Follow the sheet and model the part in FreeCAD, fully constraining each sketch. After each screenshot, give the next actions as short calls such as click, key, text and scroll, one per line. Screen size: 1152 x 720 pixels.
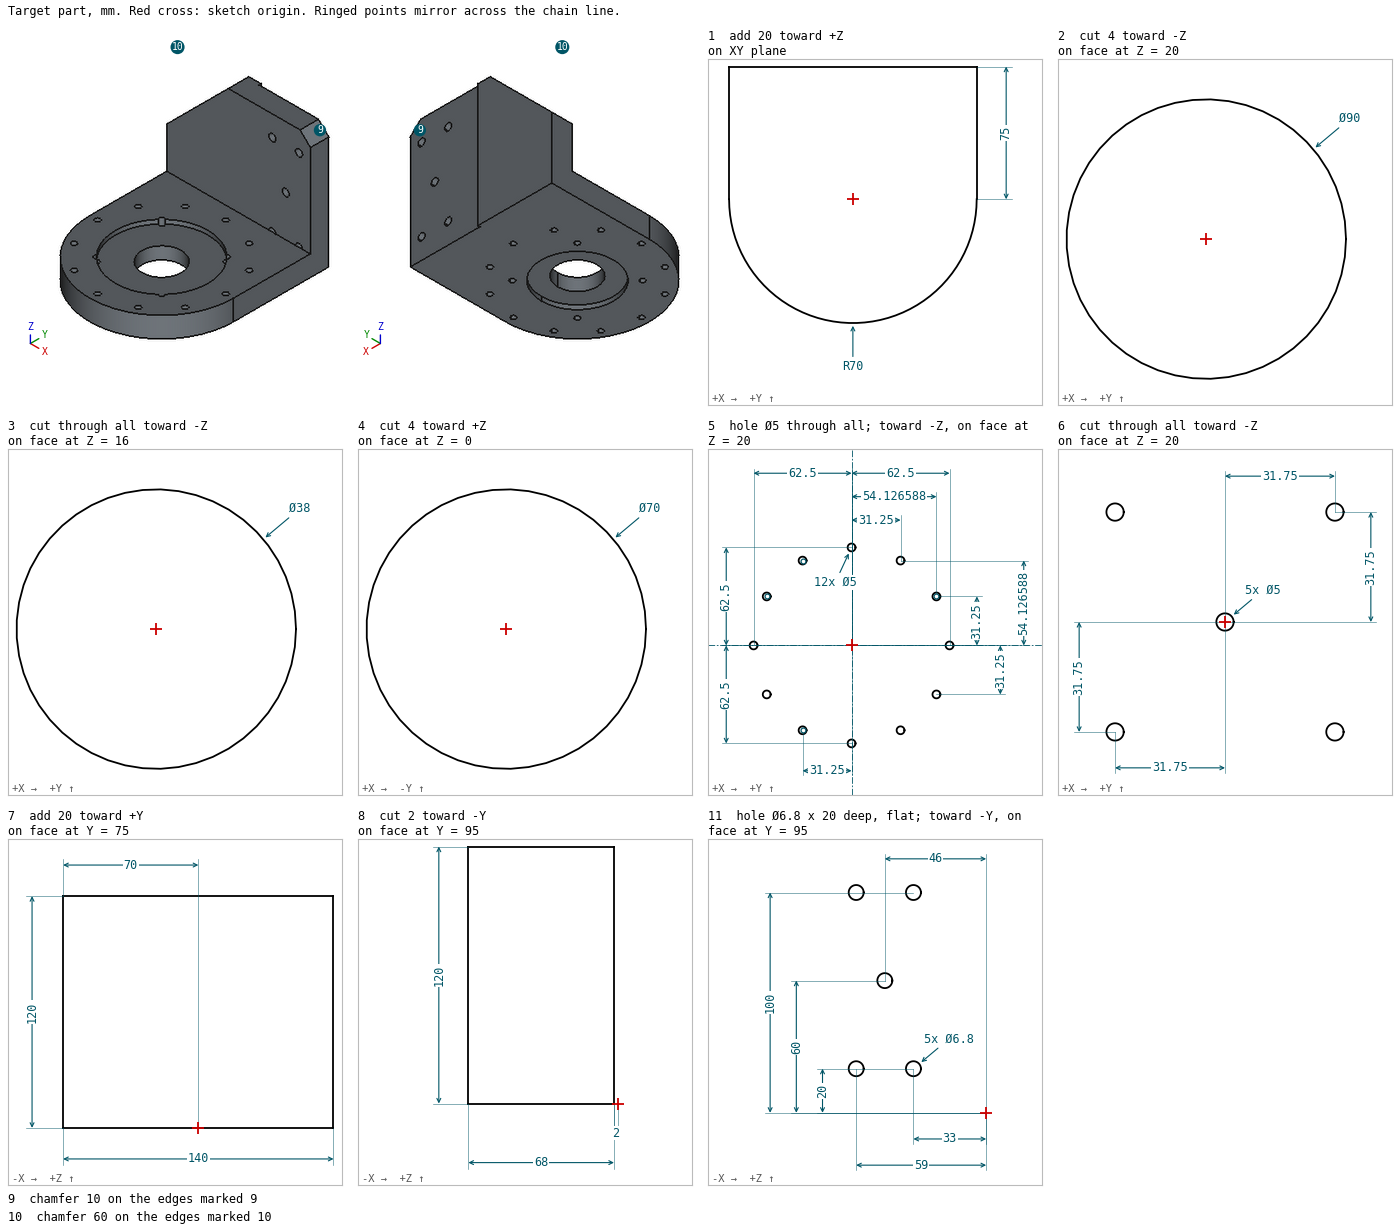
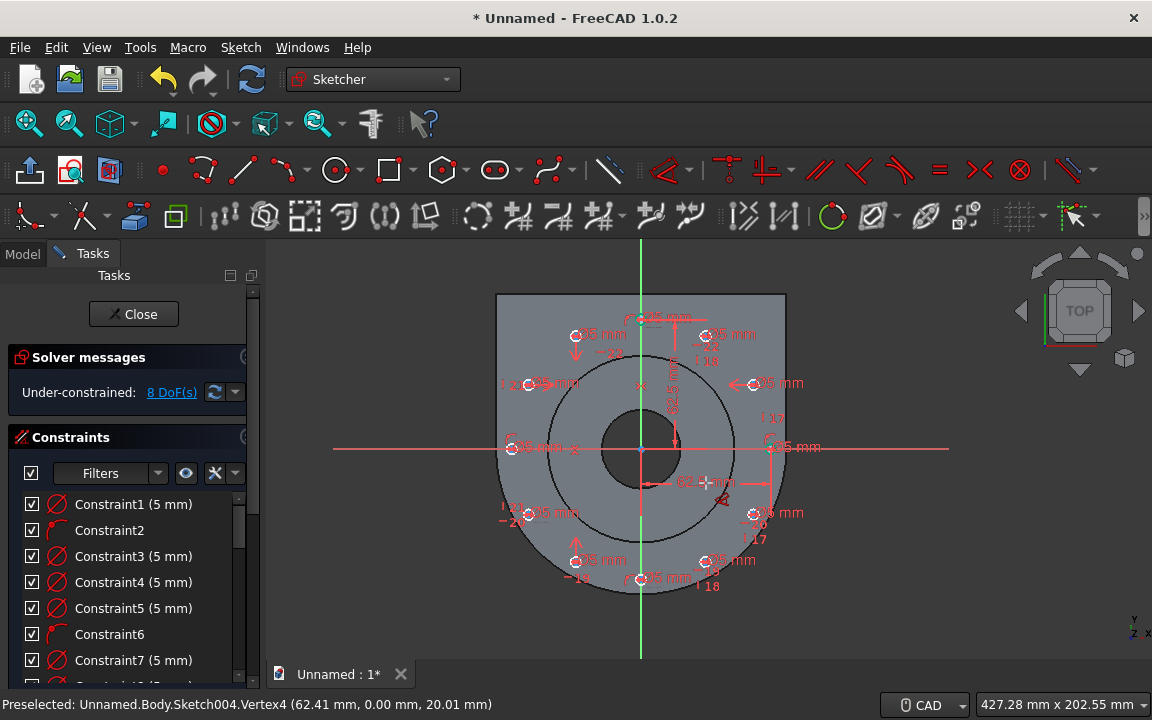
click(641, 580)
click(675, 514)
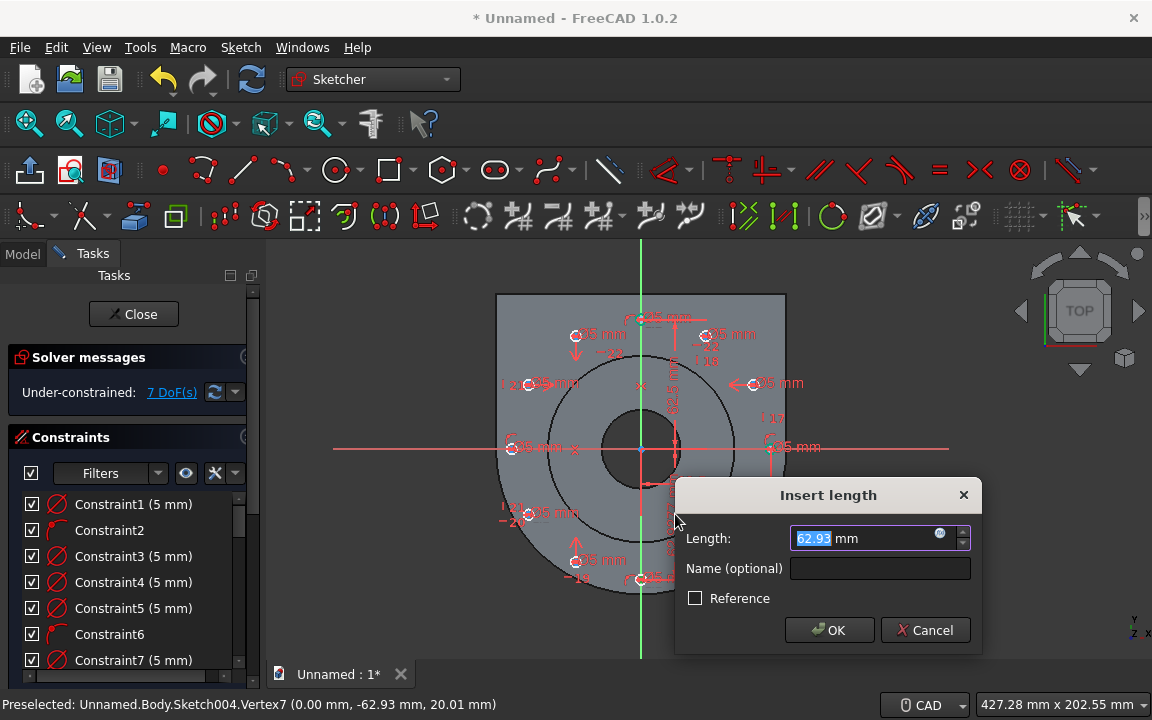
text(62.5)
key(Return)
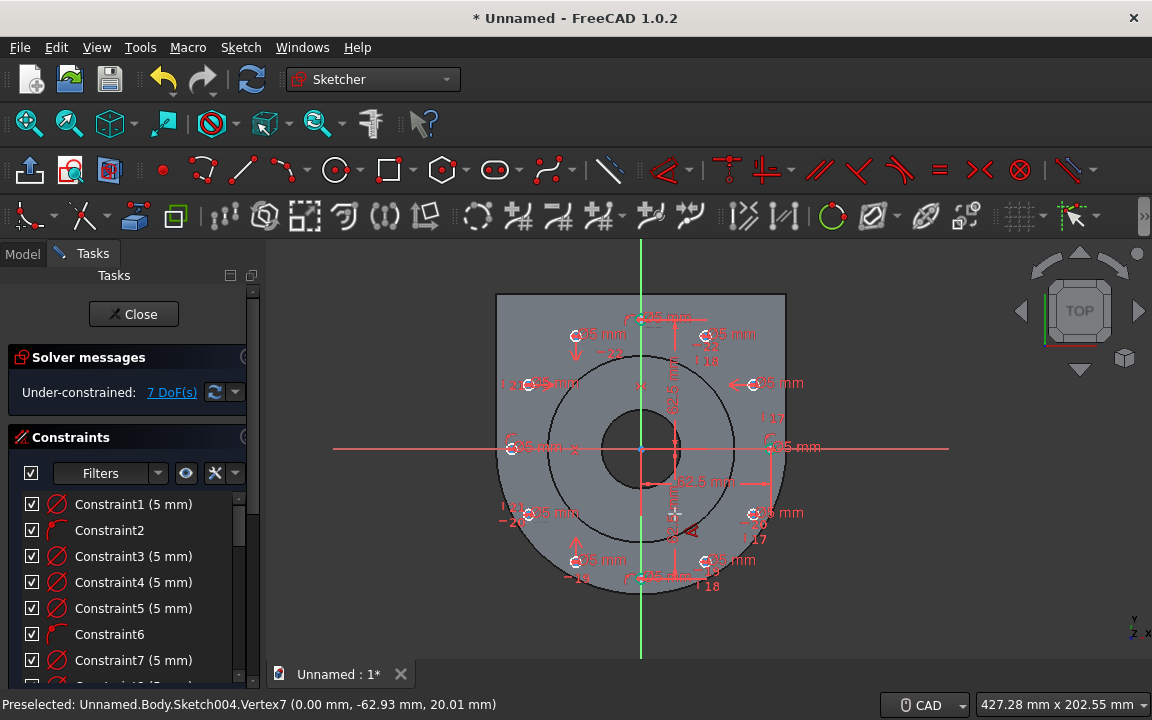
click(512, 449)
click(576, 483)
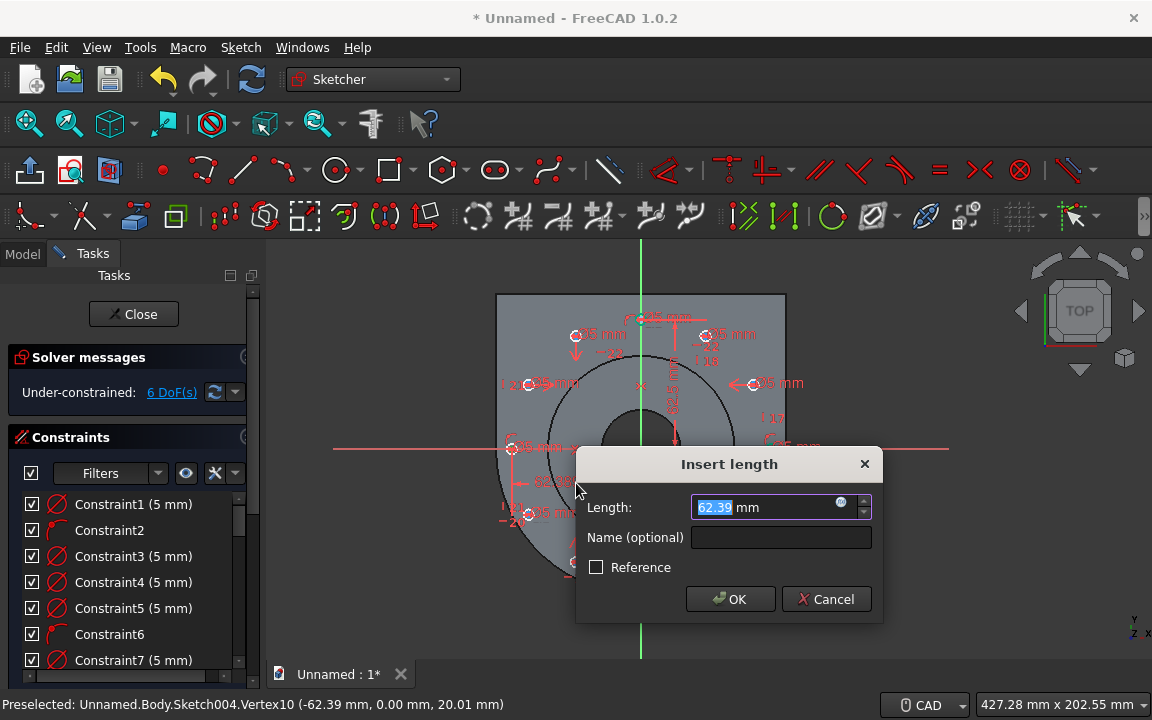
text(62.5)
key(Return)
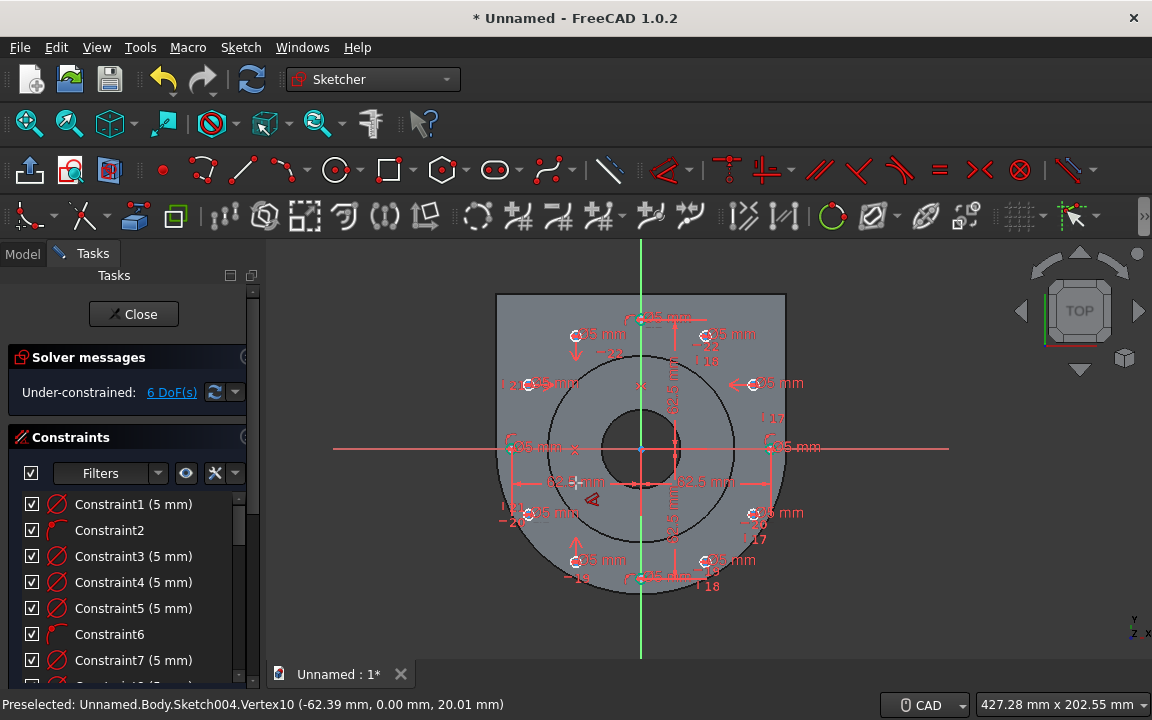
click(706, 336)
click(673, 302)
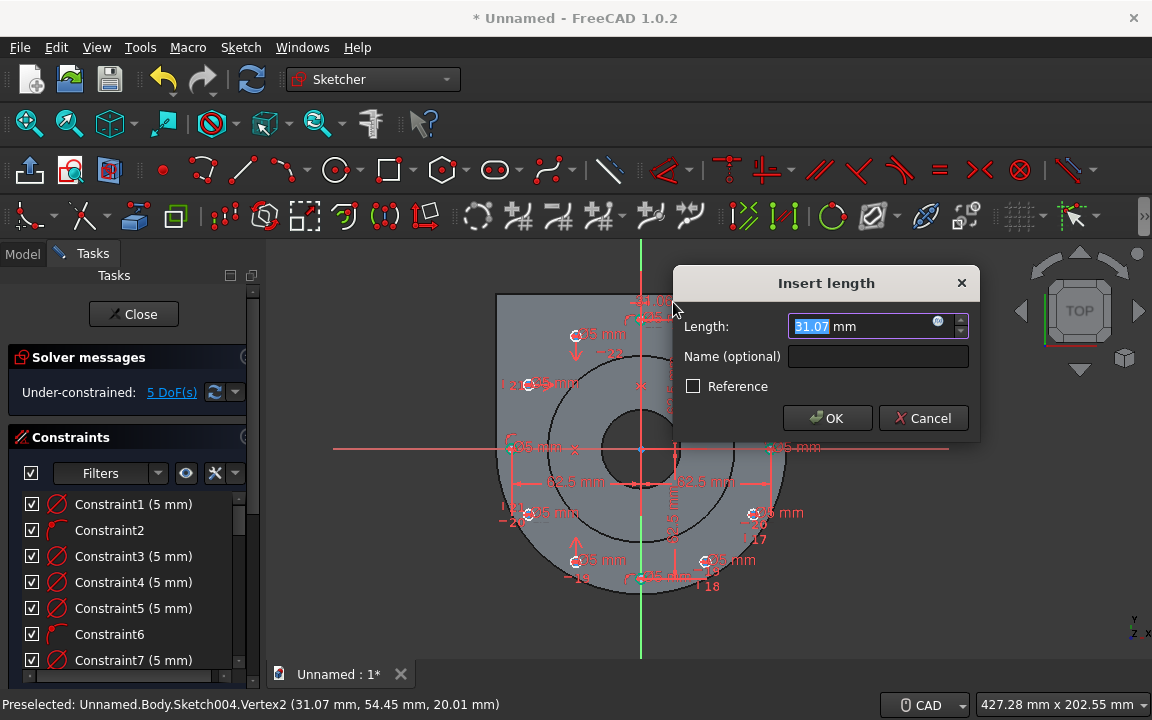
text(31.25)
key(Return)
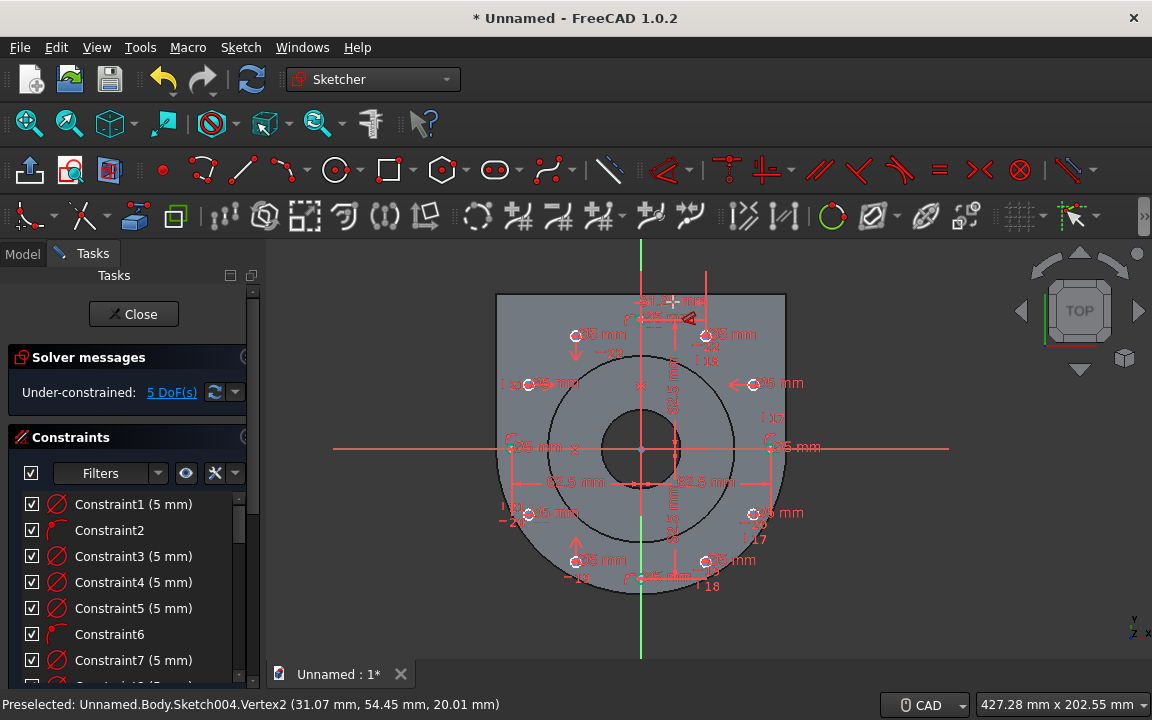
click(754, 385)
click(788, 417)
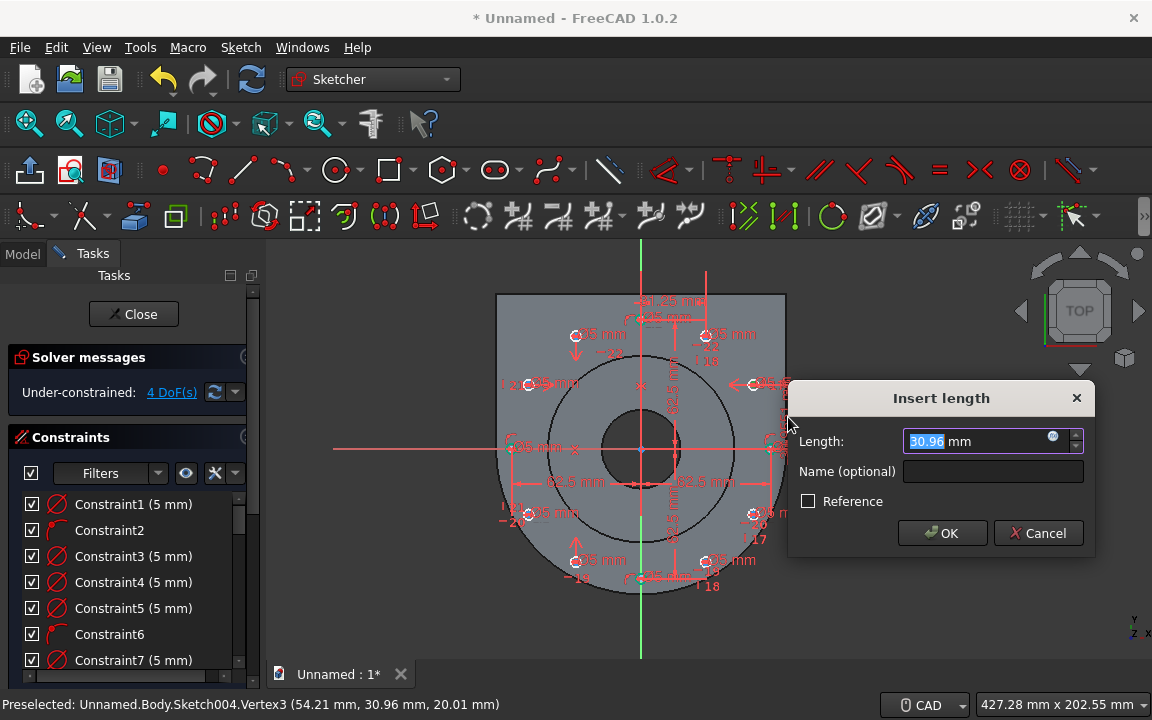
text(31.25)
key(Return)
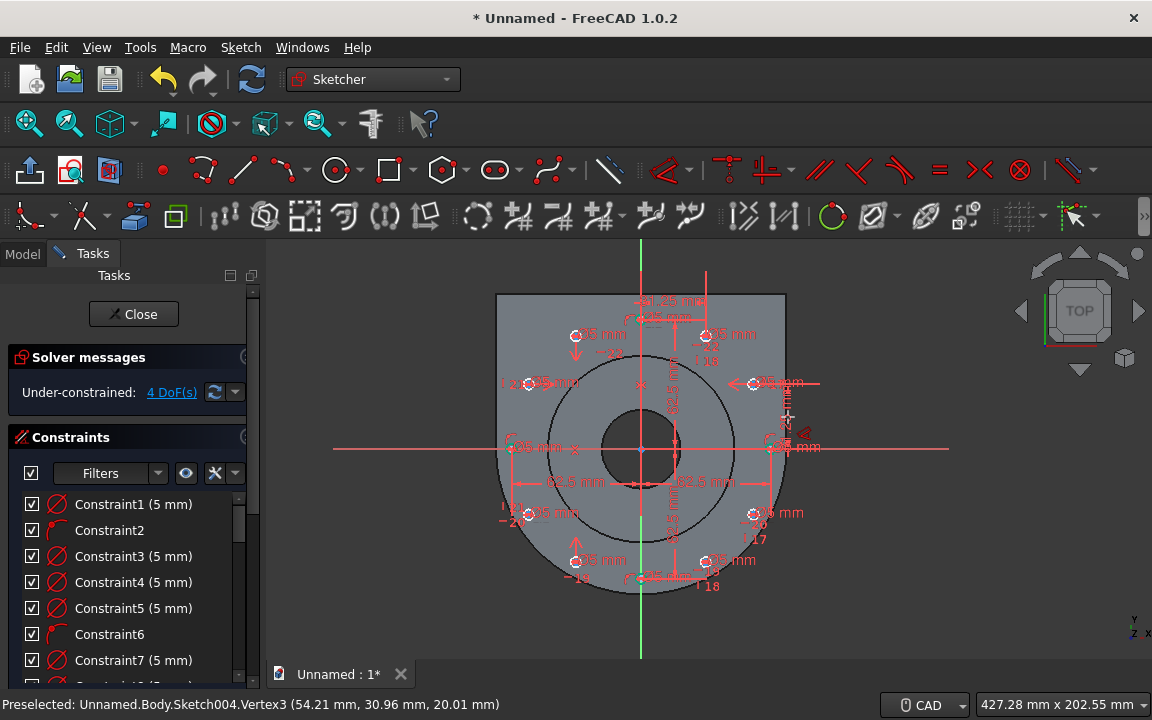
click(754, 515)
click(788, 482)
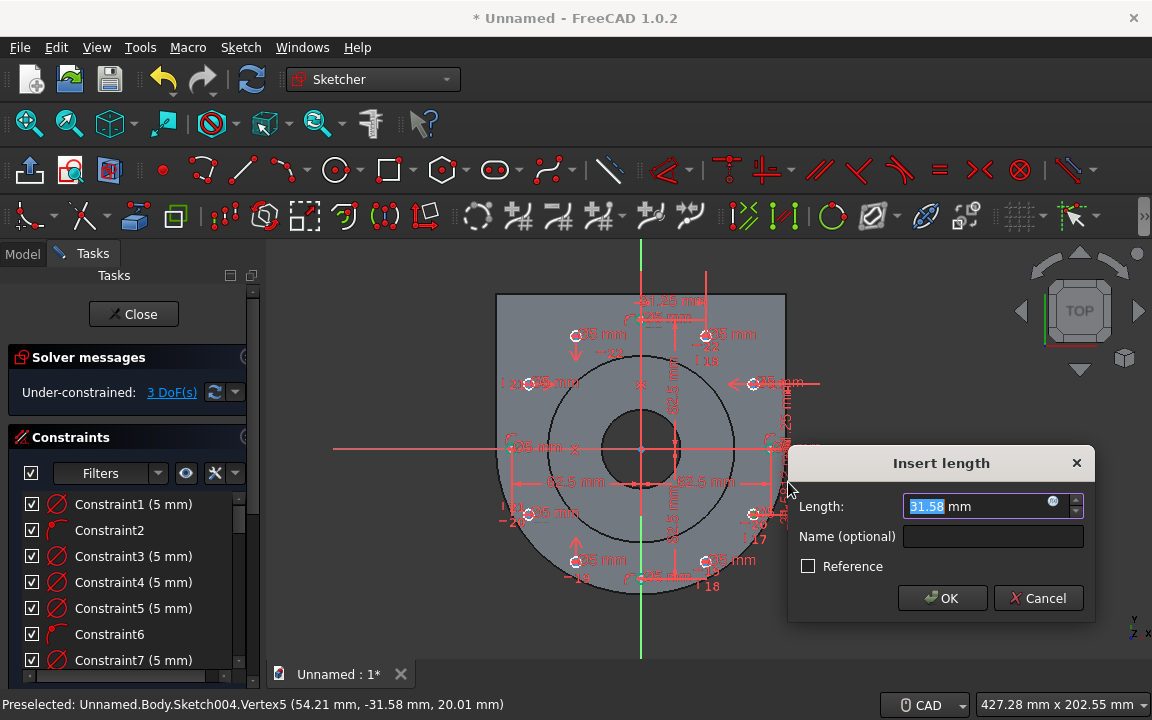
text(31.25)
key(Return)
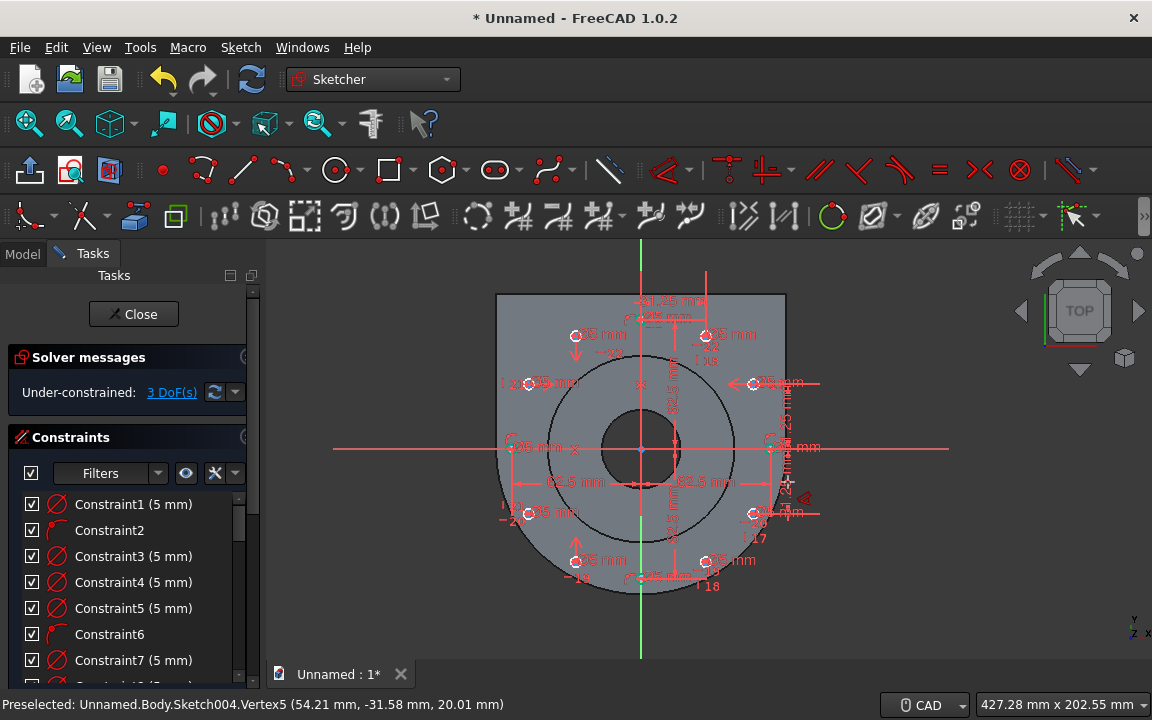
click(576, 562)
click(609, 596)